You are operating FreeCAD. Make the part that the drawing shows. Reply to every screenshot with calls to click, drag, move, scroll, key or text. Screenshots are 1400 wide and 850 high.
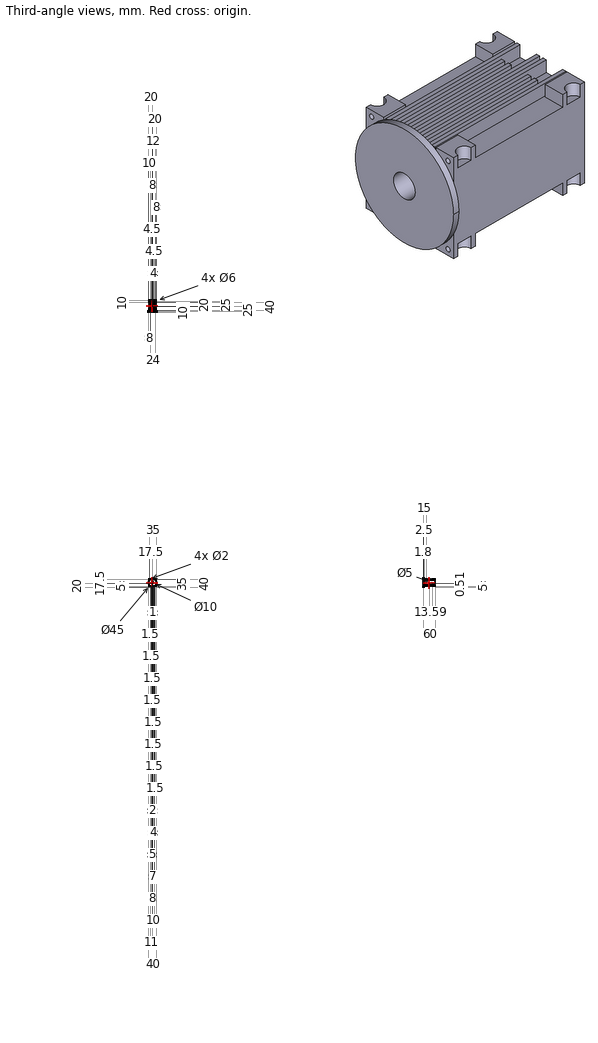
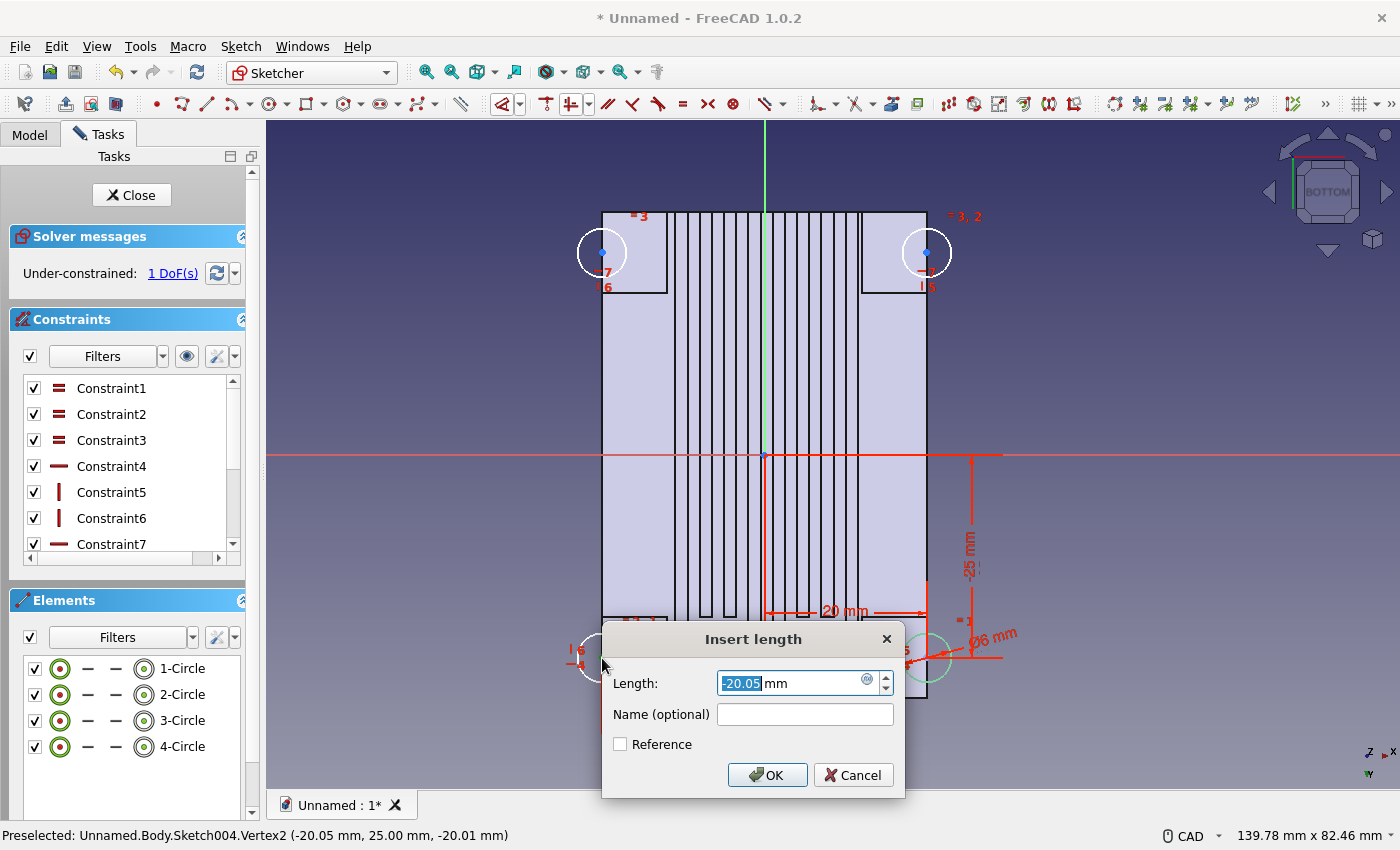
text(-20)
key(Return)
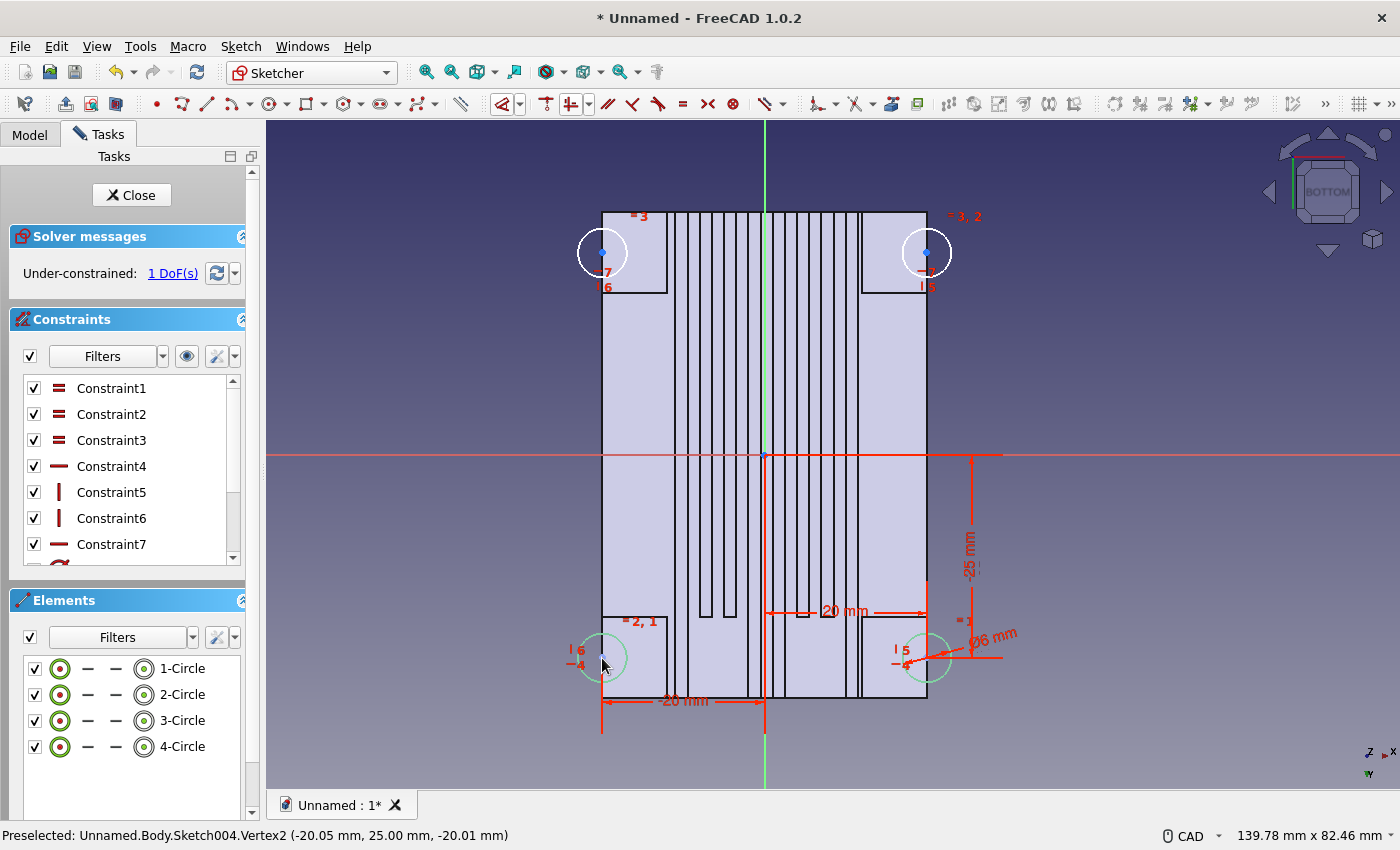
click(927, 253)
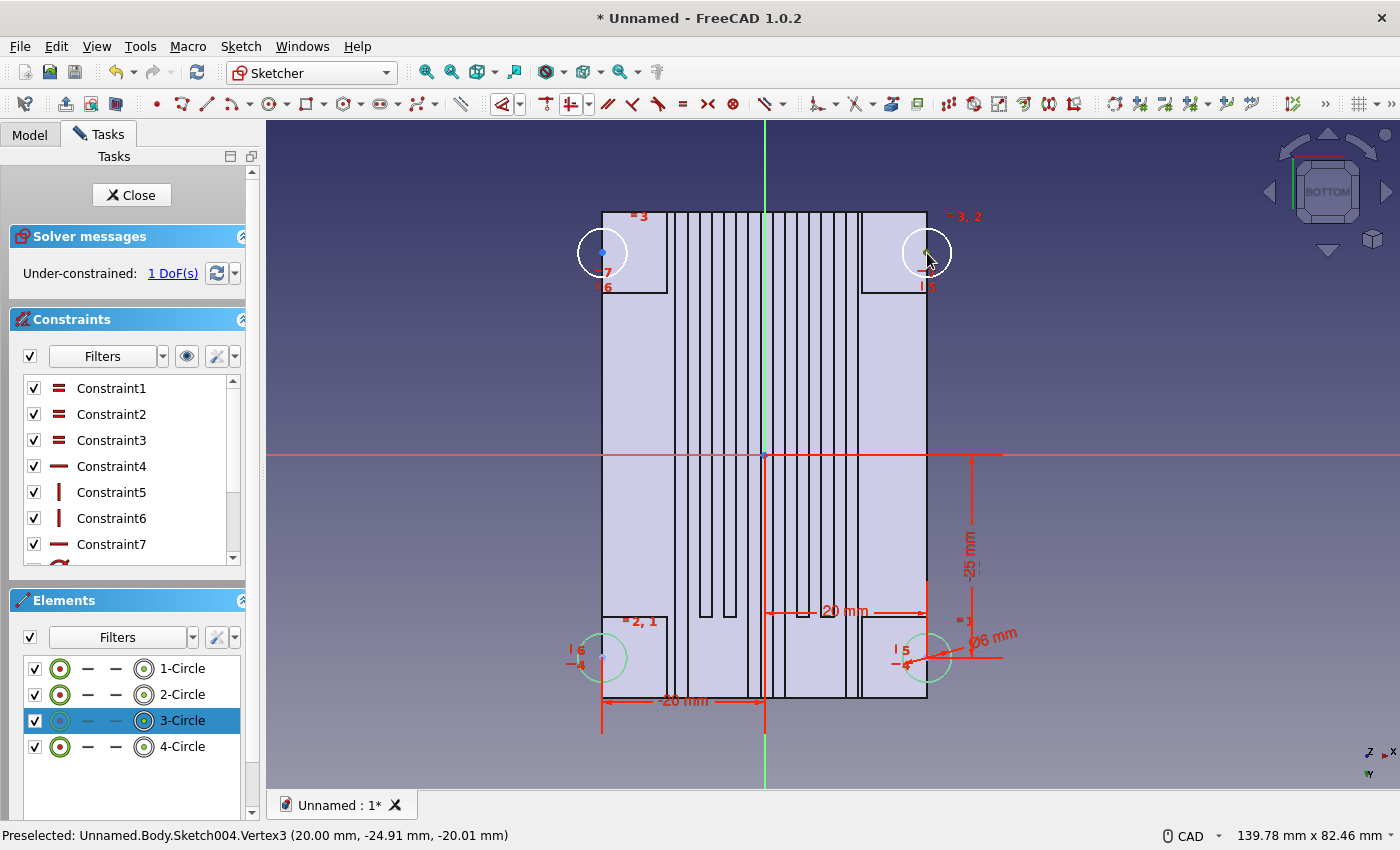
click(520, 104)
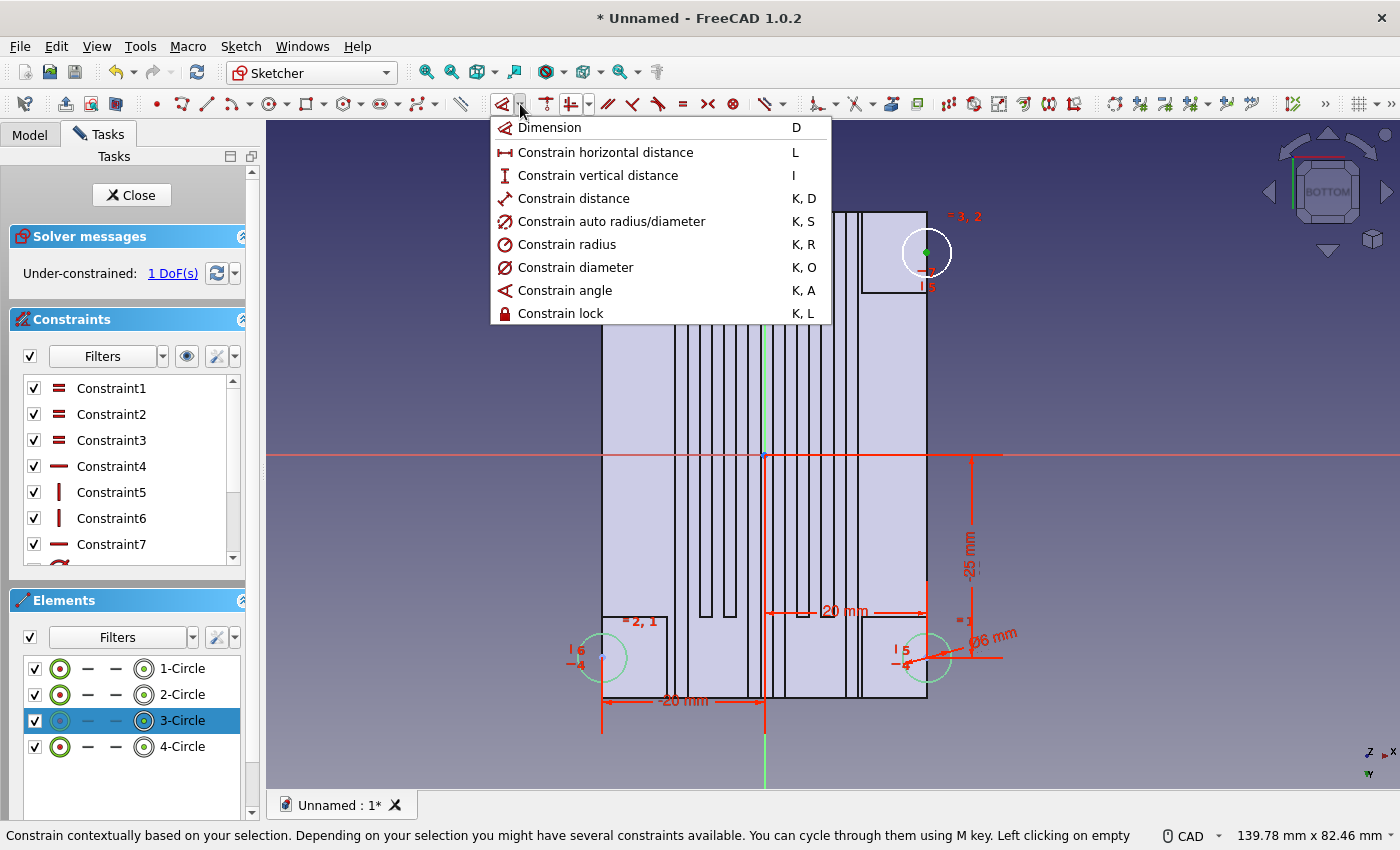
click(661, 176)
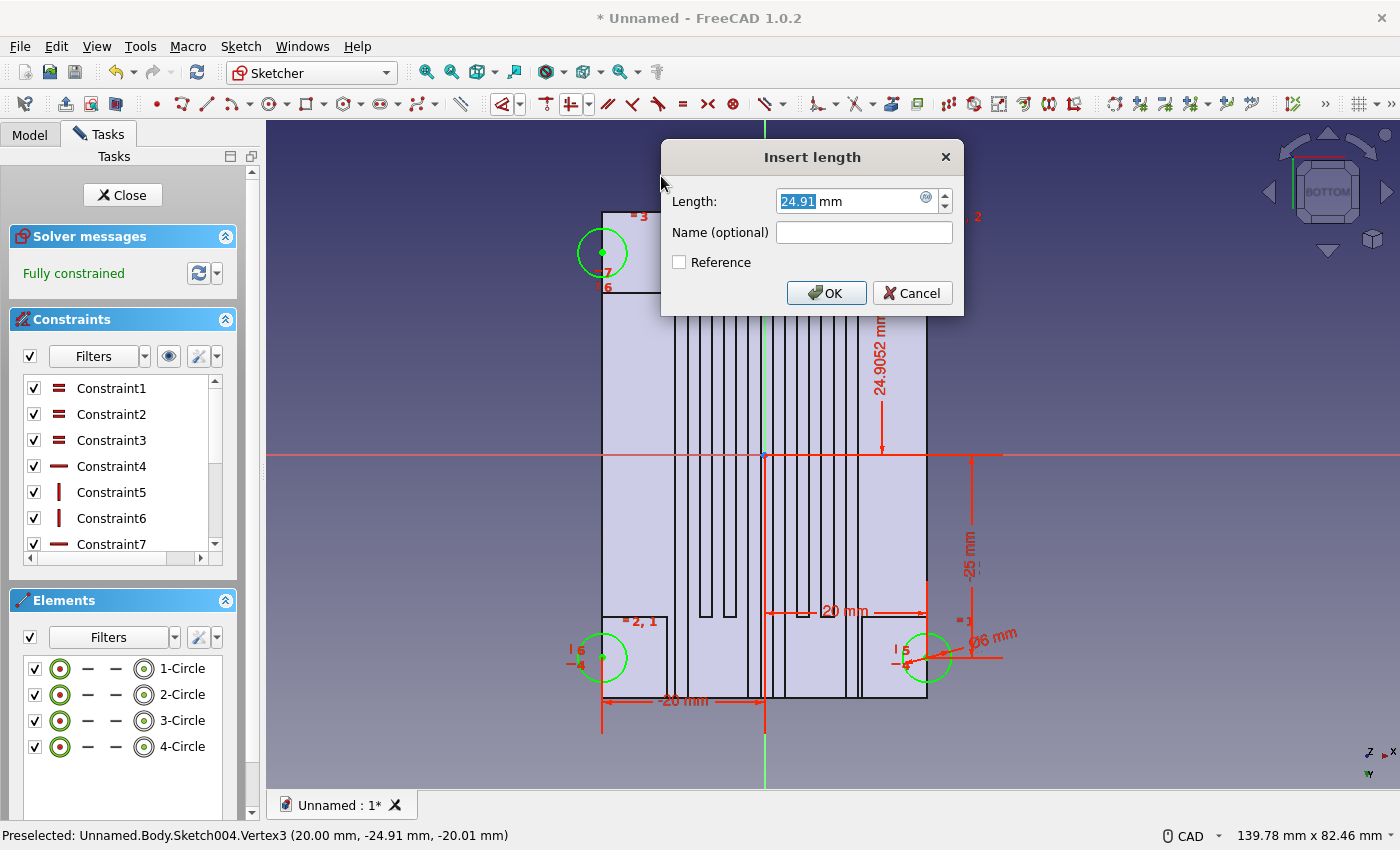
text(25)
key(Return)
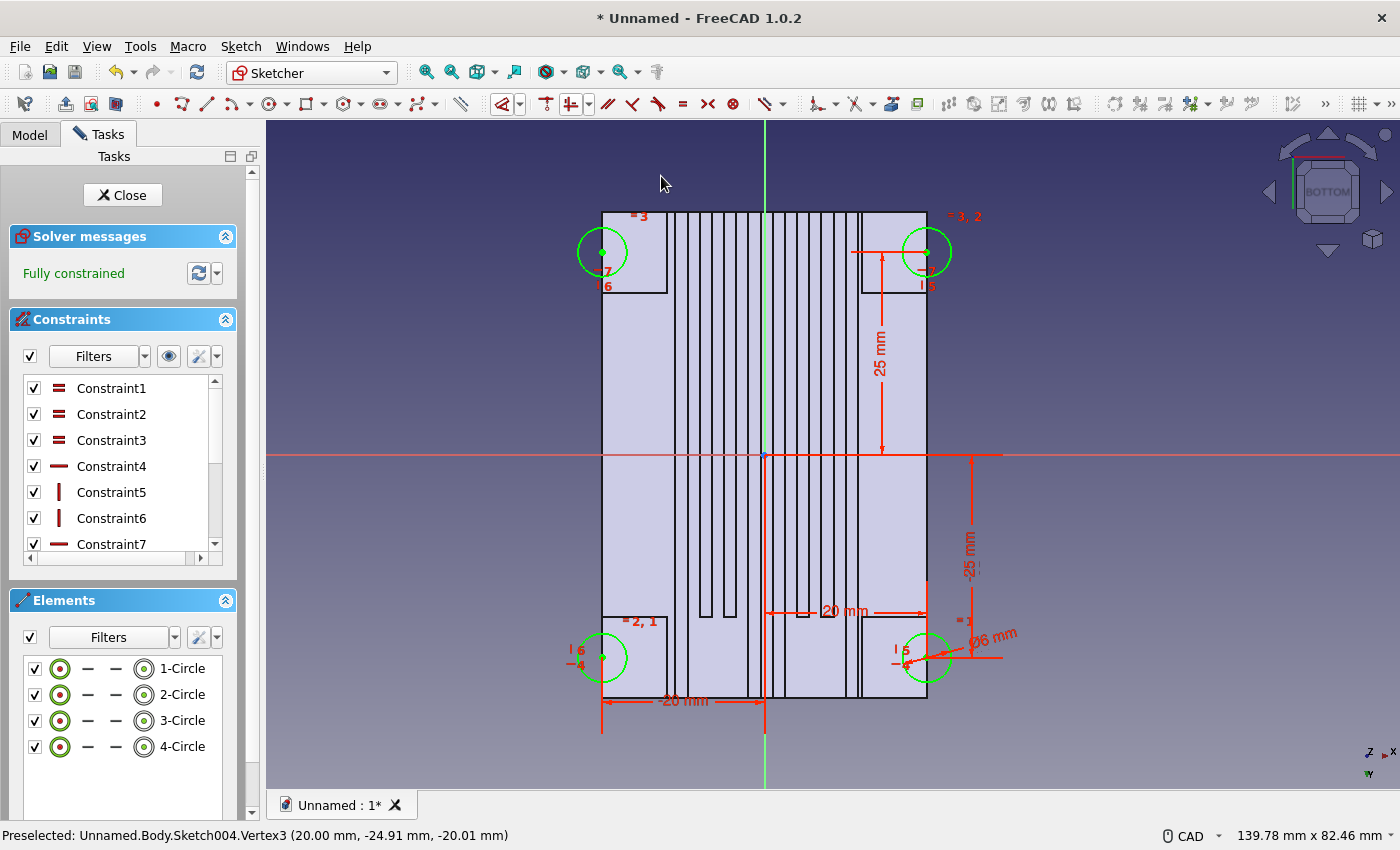
click(123, 195)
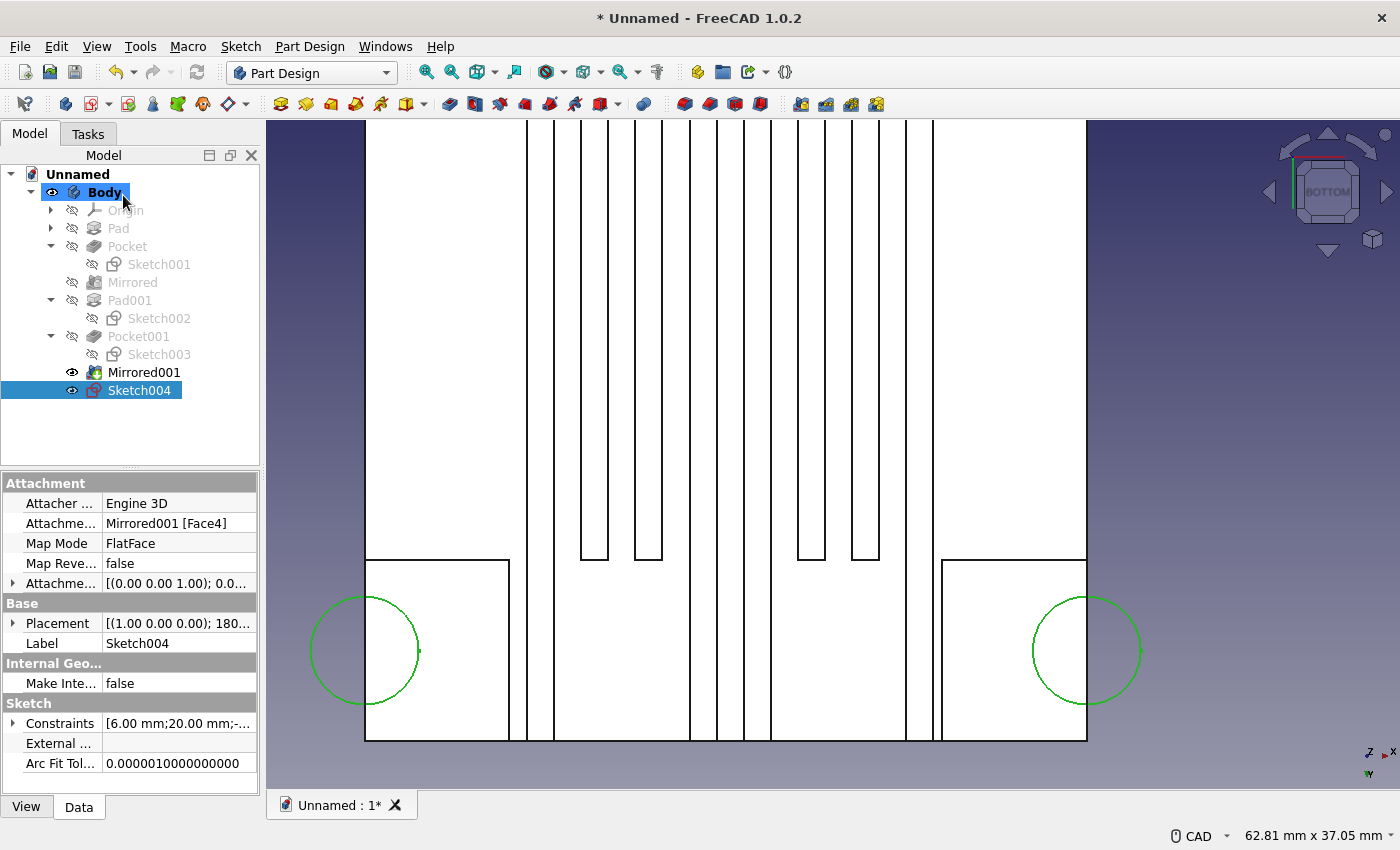
click(450, 104)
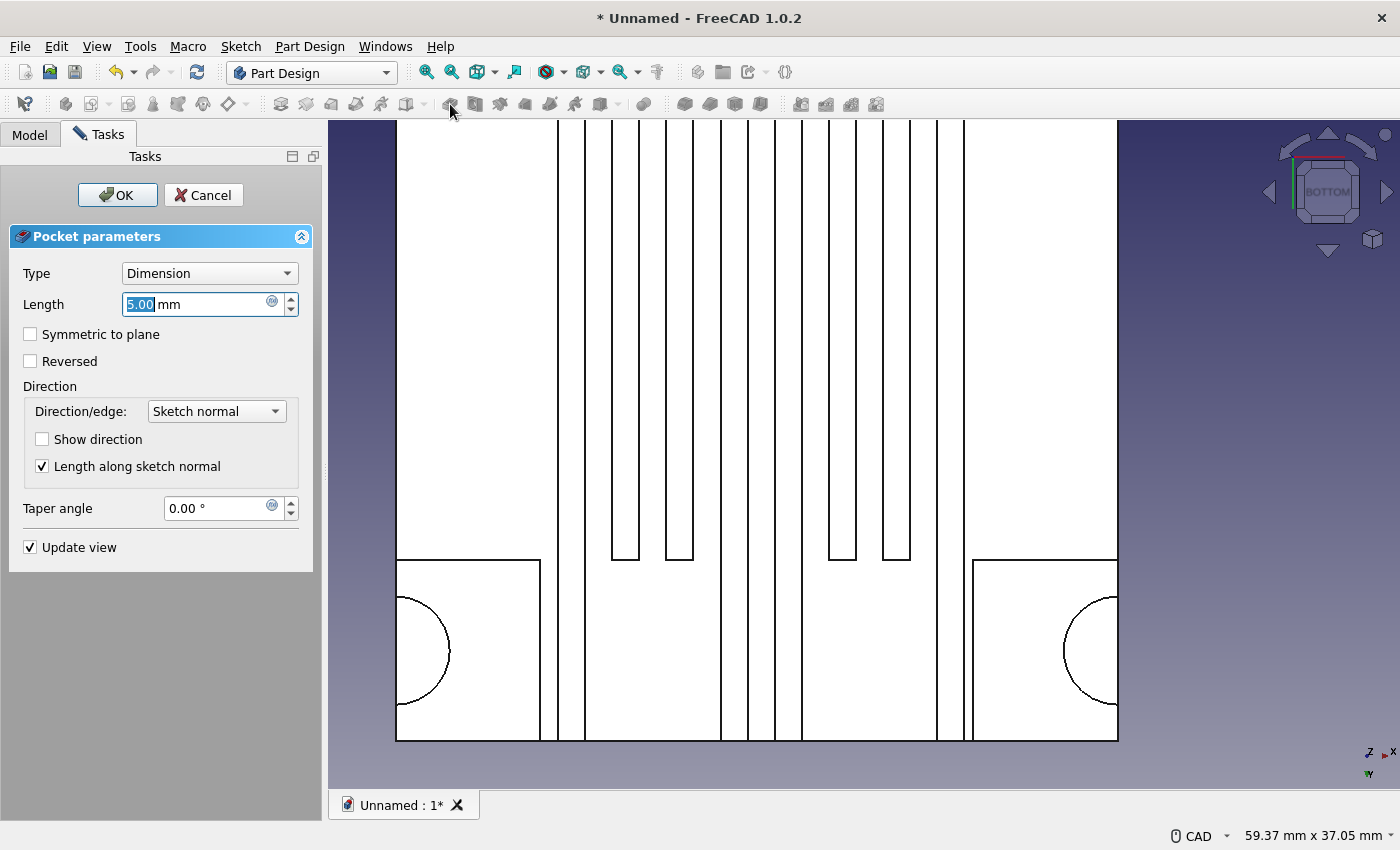
text(5)
key(Tab)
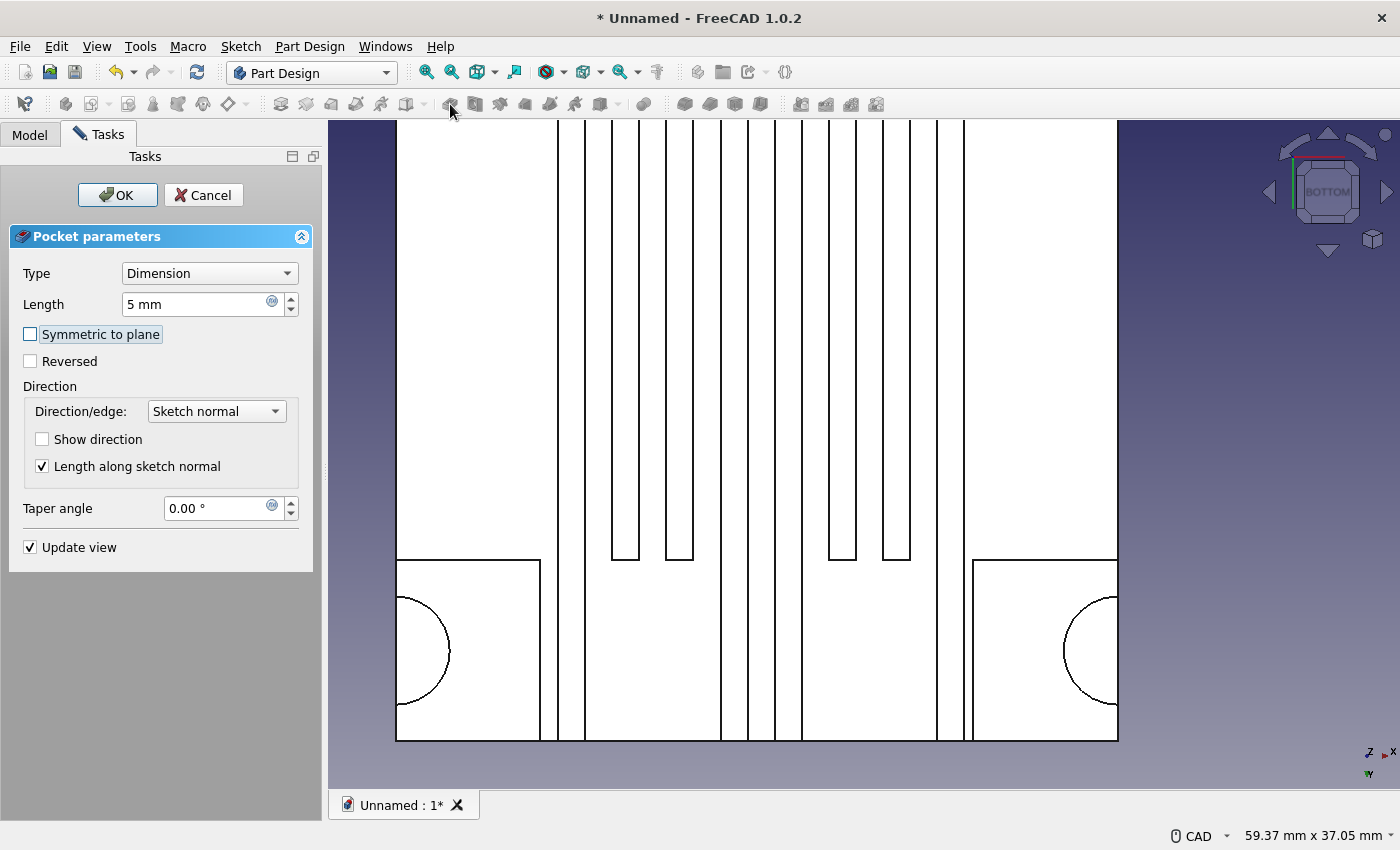
click(118, 195)